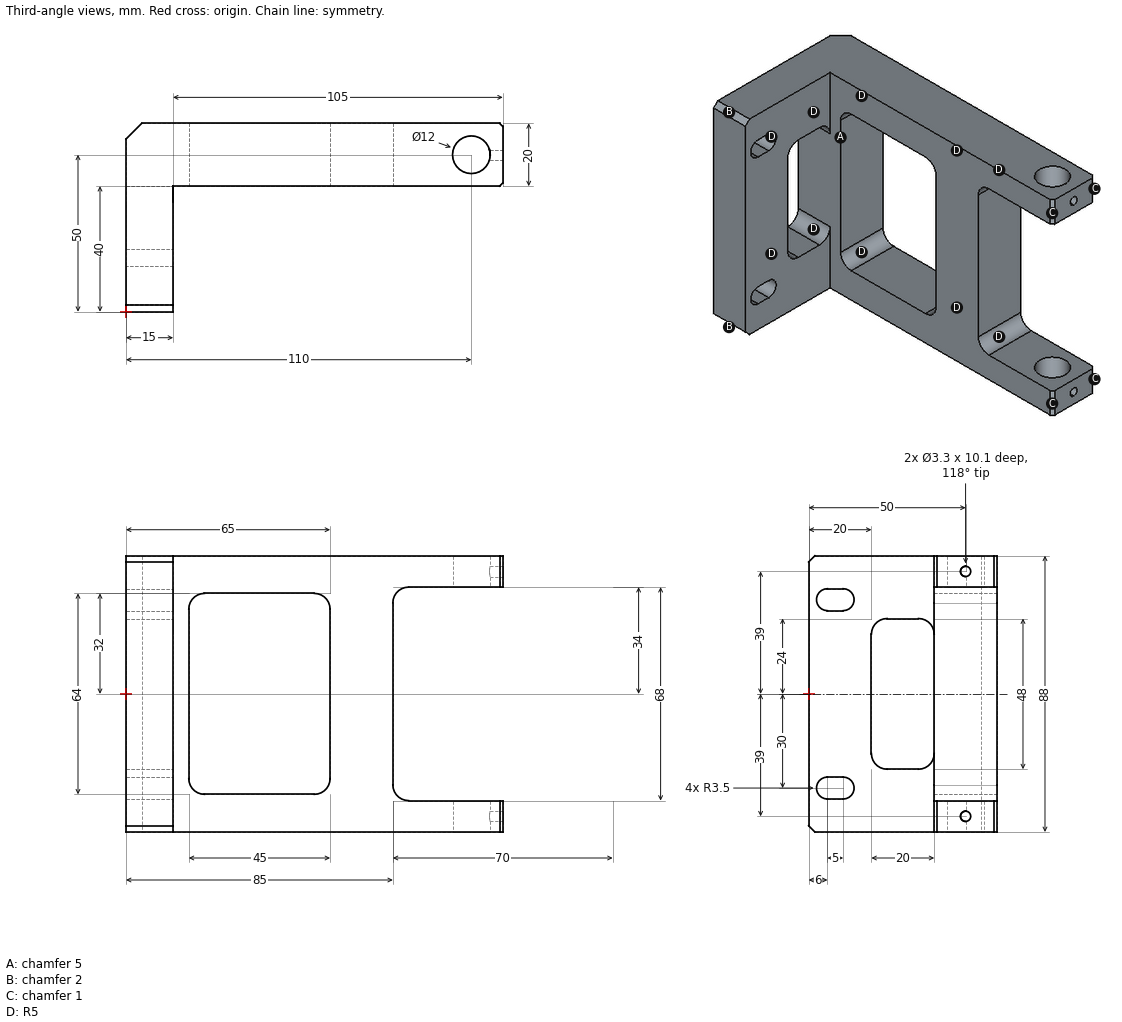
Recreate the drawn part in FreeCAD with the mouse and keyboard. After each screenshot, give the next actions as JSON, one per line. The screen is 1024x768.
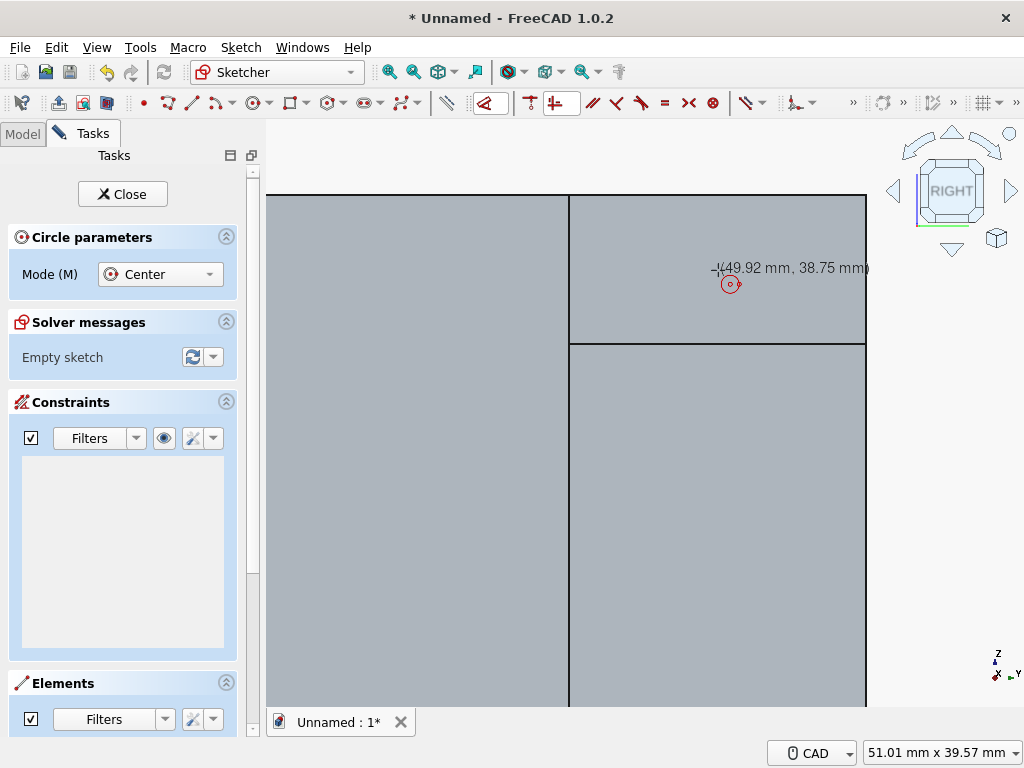
{"action": "scroll", "coordinate": [671, 225], "scroll_direction": "down", "scroll_amount": 6}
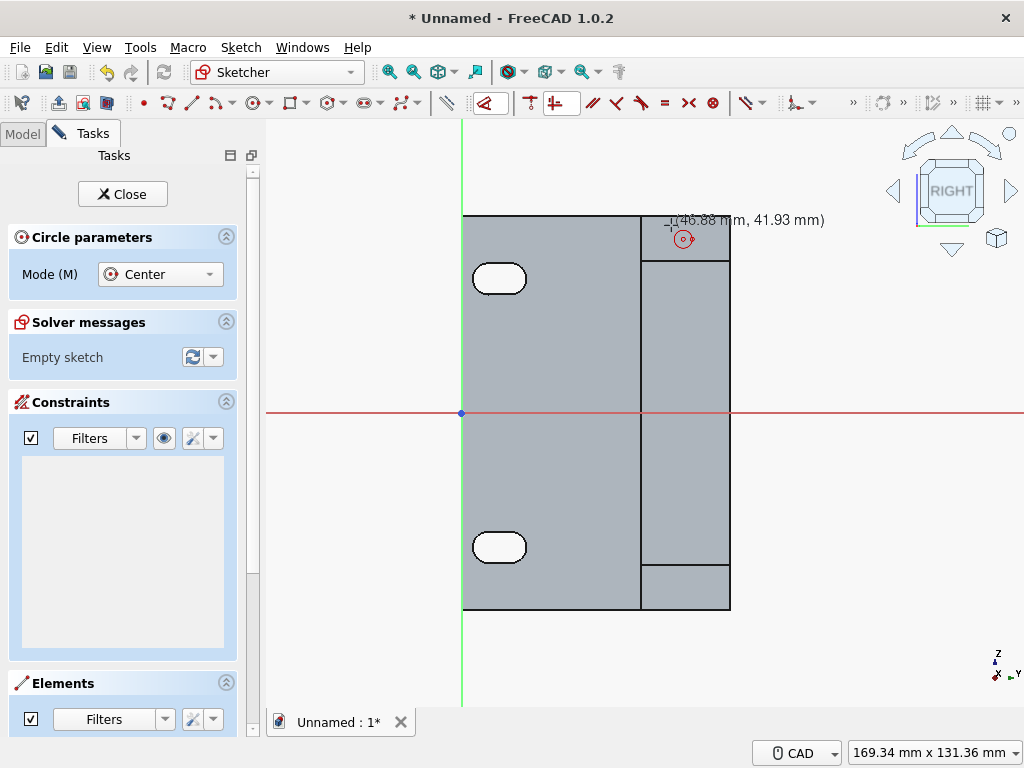
{"action": "left_click", "coordinate": [685, 239]}
{"action": "mouse_move", "coordinate": [691, 233]}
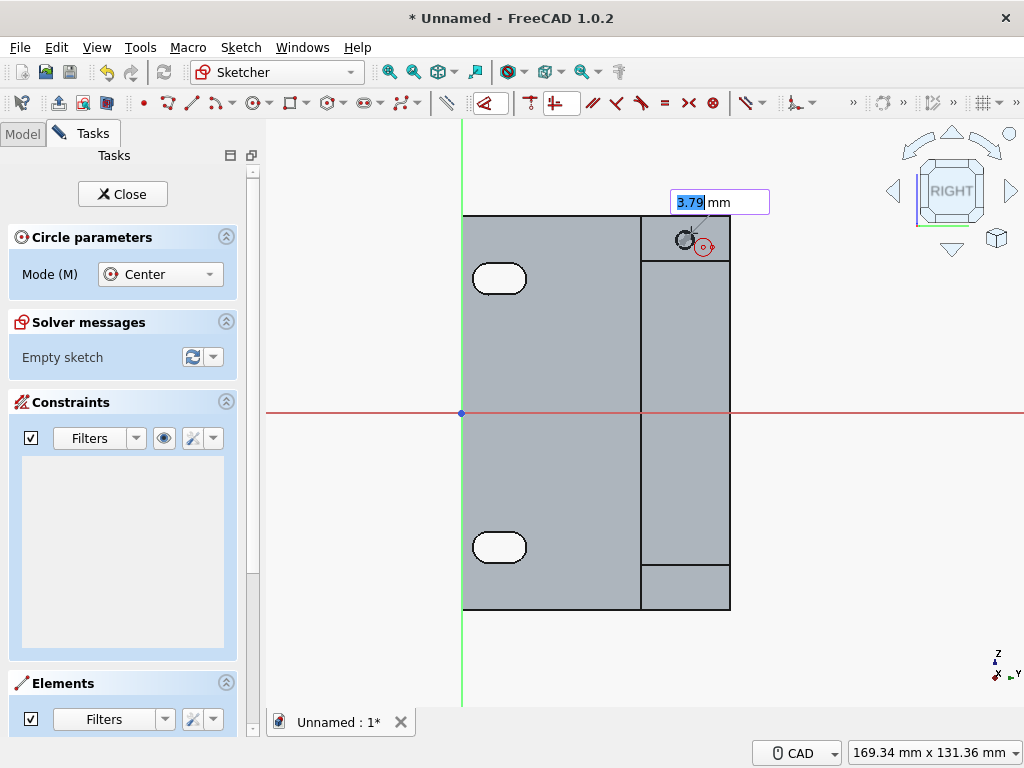
{"action": "type", "text": "3.3"}
{"action": "key", "text": "Return"}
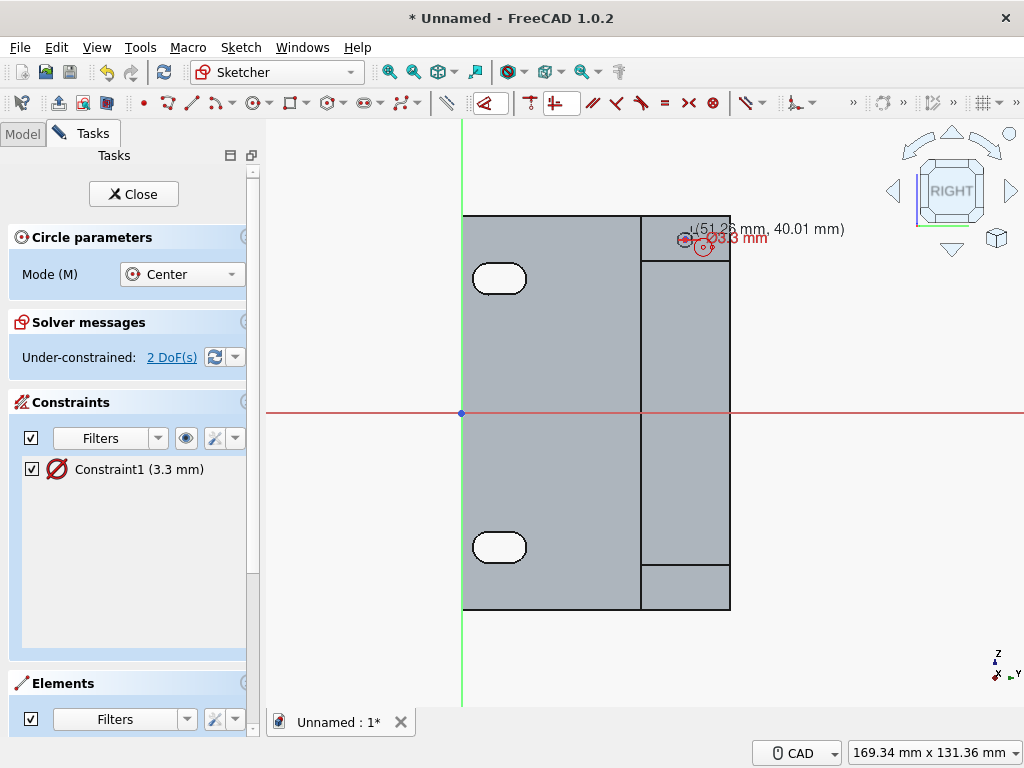
{"action": "scroll", "coordinate": [685, 588], "scroll_direction": "up", "scroll_amount": 6}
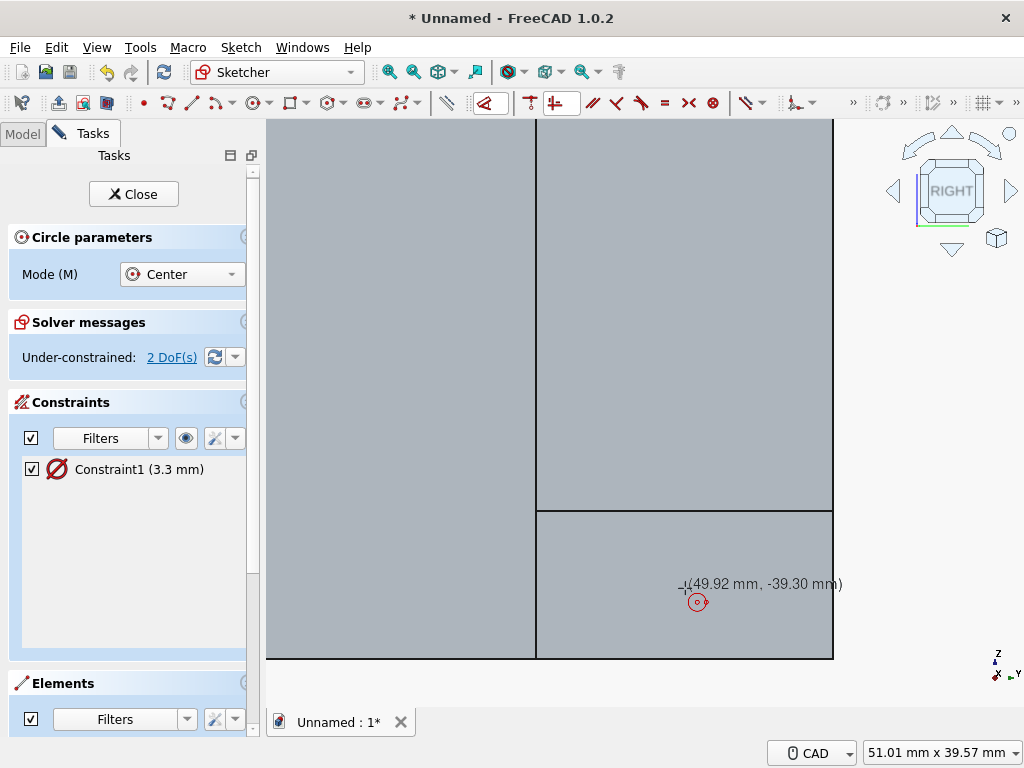
{"action": "scroll", "coordinate": [685, 589], "scroll_direction": "down", "scroll_amount": 6}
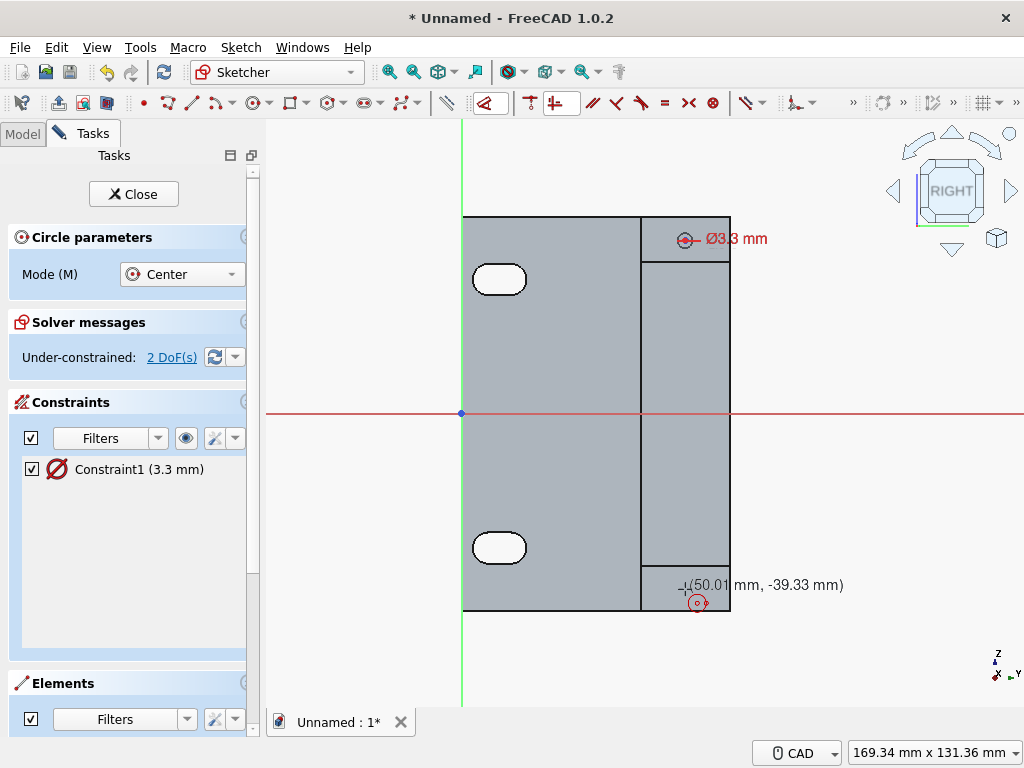
{"action": "left_click", "coordinate": [685, 588]}
{"action": "mouse_move", "coordinate": [691, 583]}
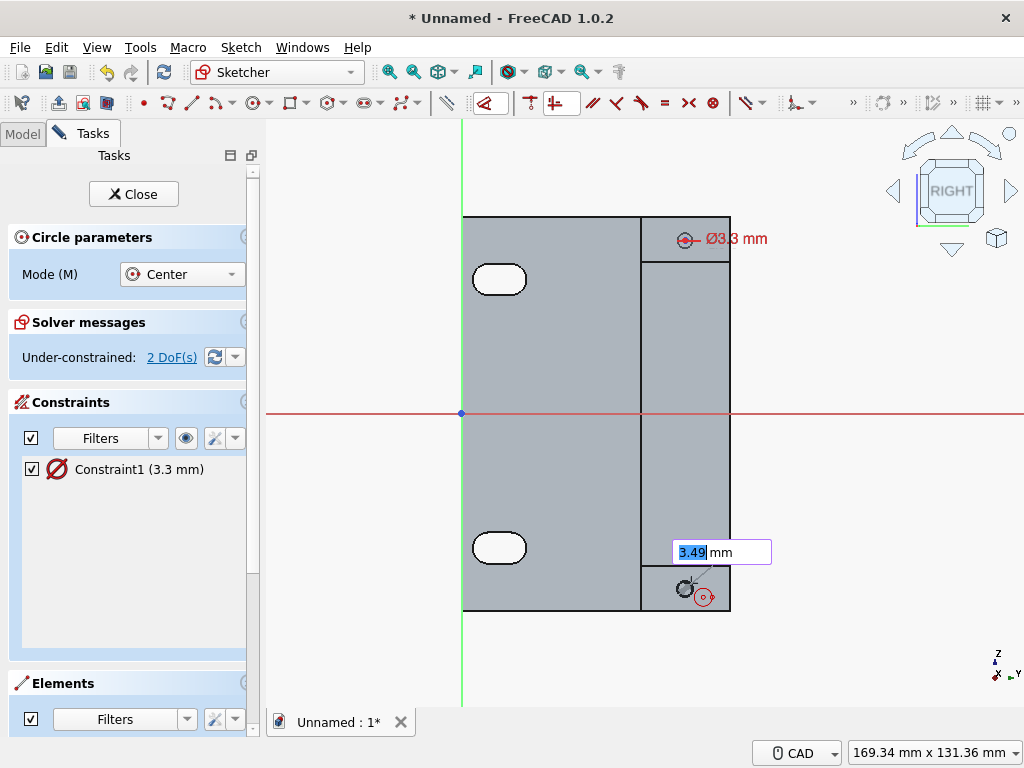
{"action": "type", "text": "3.3"}
{"action": "key", "text": "Return"}
{"action": "key", "text": "Escape"}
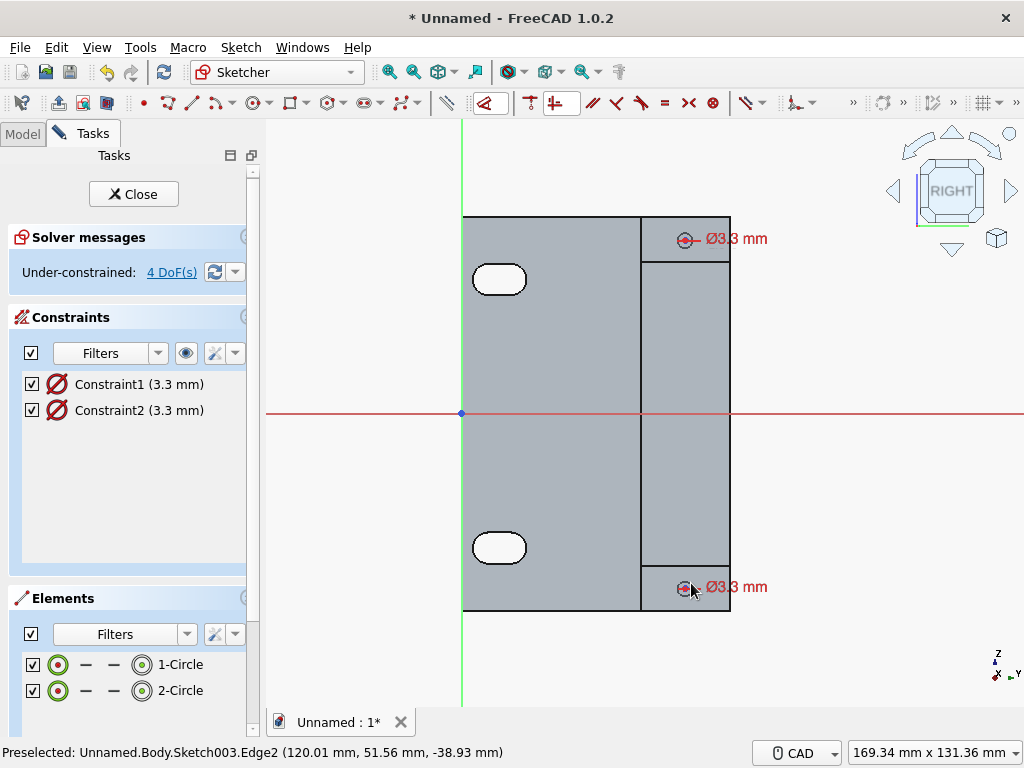
{"action": "left_click", "coordinate": [685, 241]}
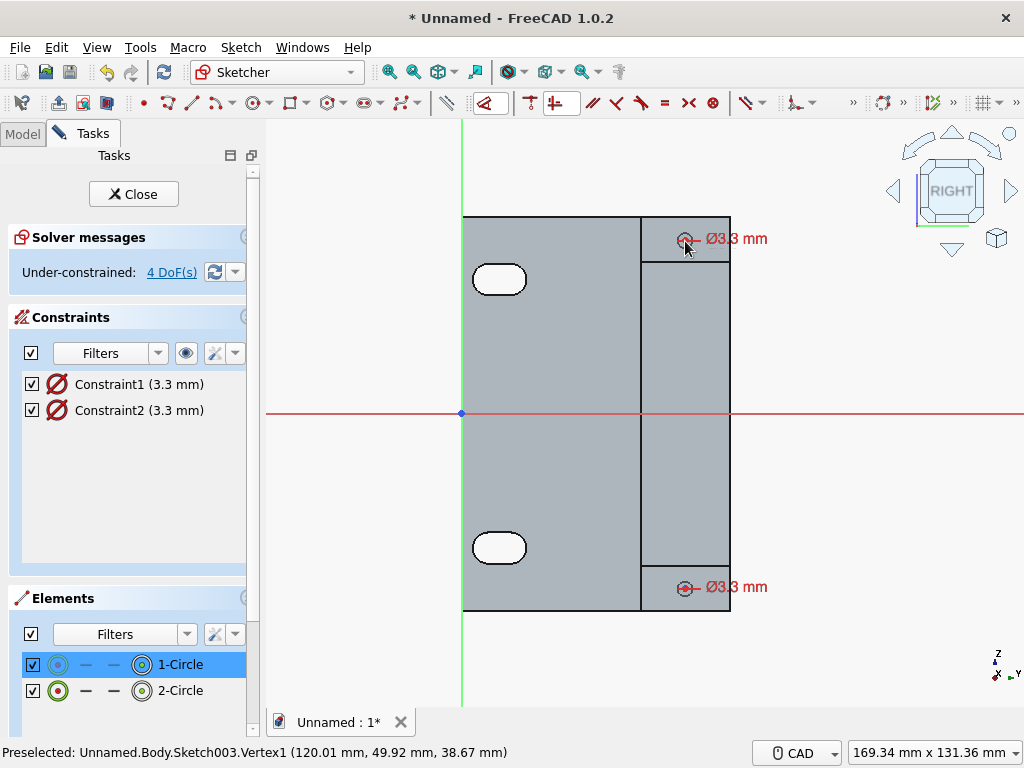
{"action": "left_click", "coordinate": [685, 589]}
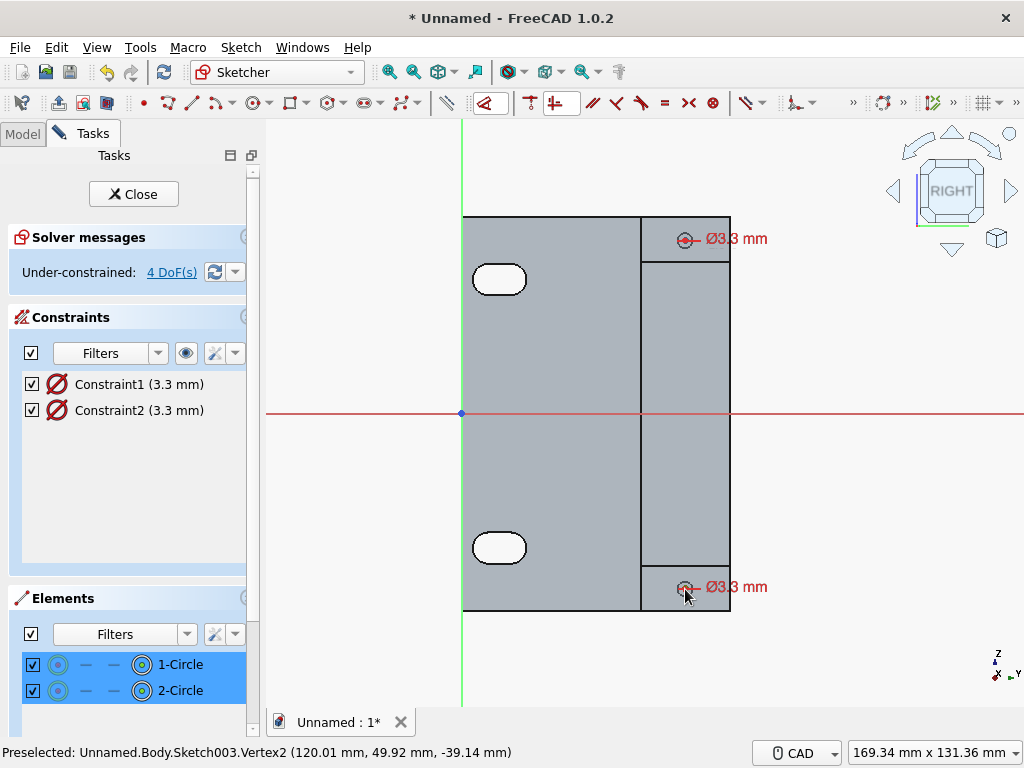
{"action": "key", "text": "v"}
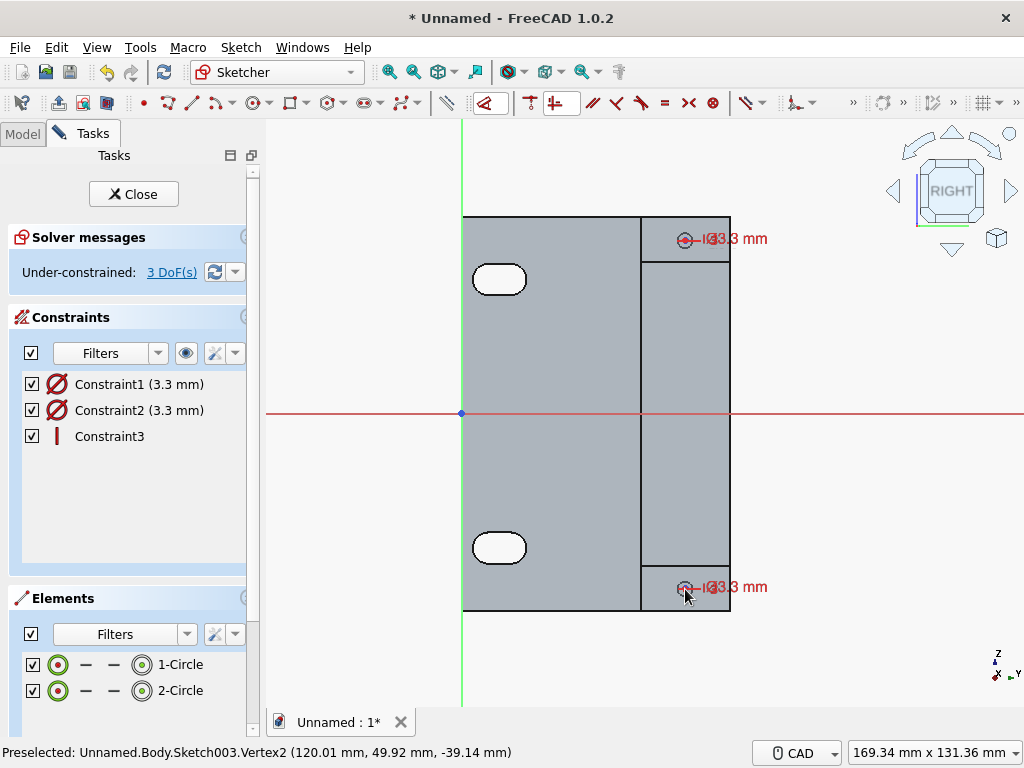
{"action": "left_click", "coordinate": [685, 241]}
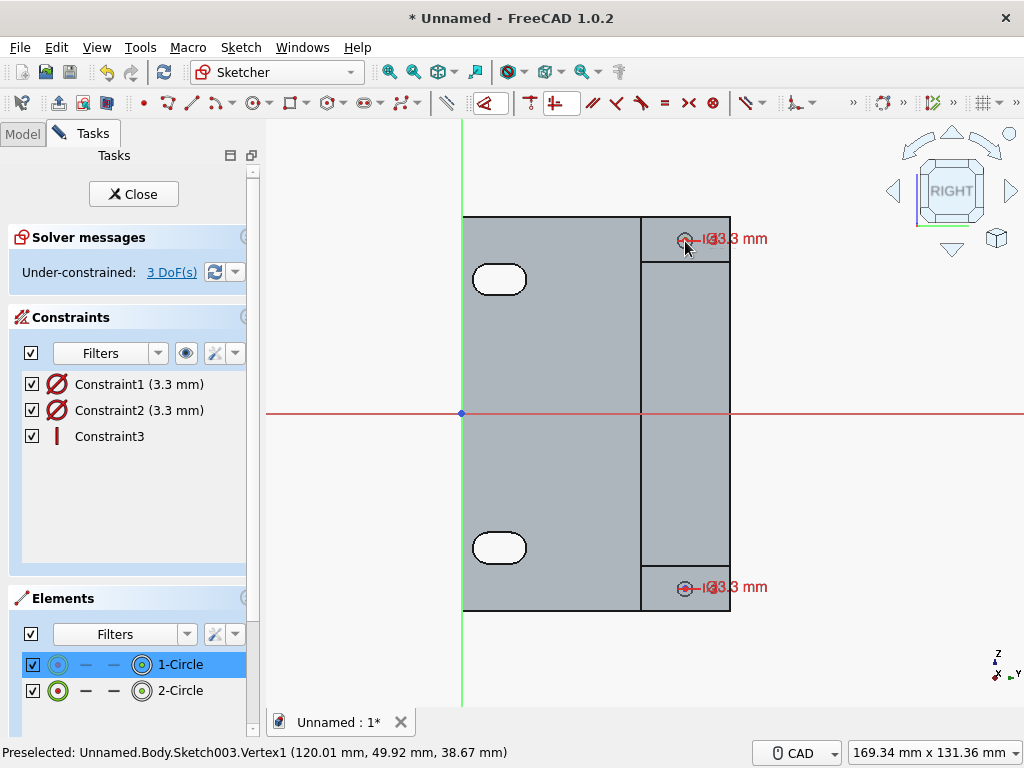
{"action": "key", "text": "l"}